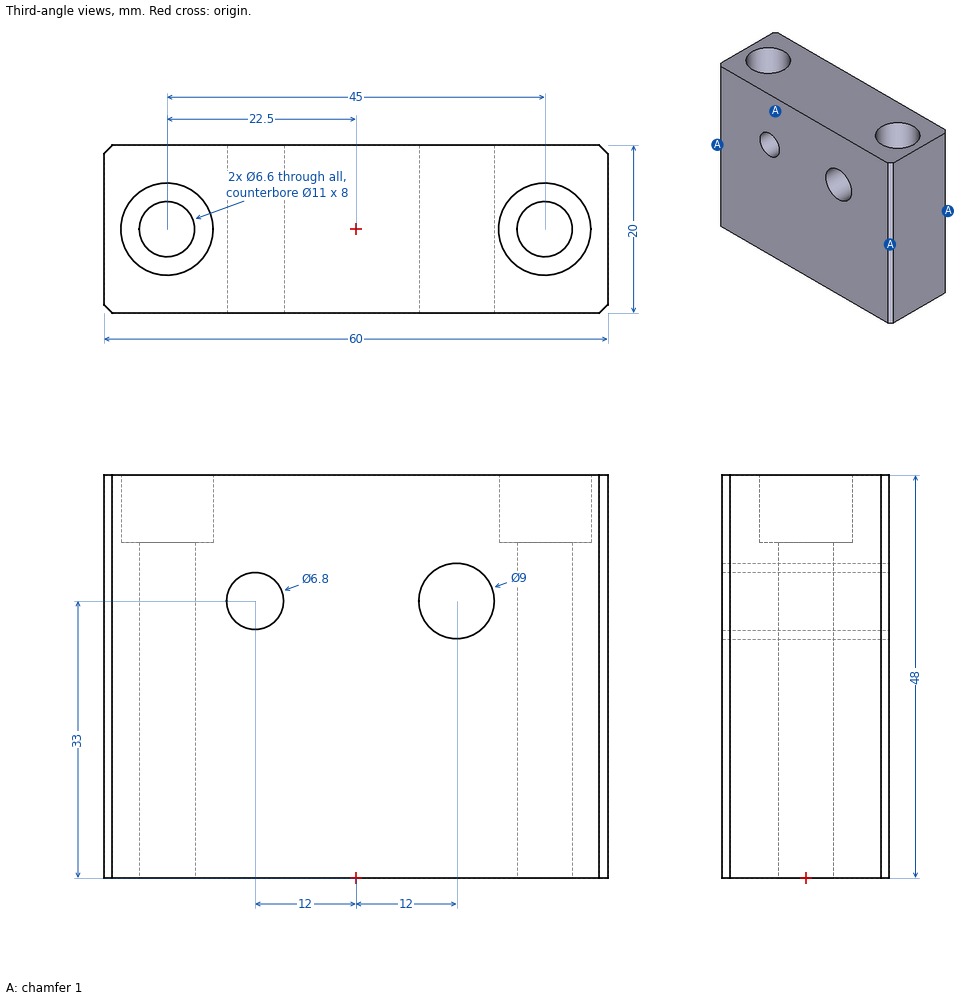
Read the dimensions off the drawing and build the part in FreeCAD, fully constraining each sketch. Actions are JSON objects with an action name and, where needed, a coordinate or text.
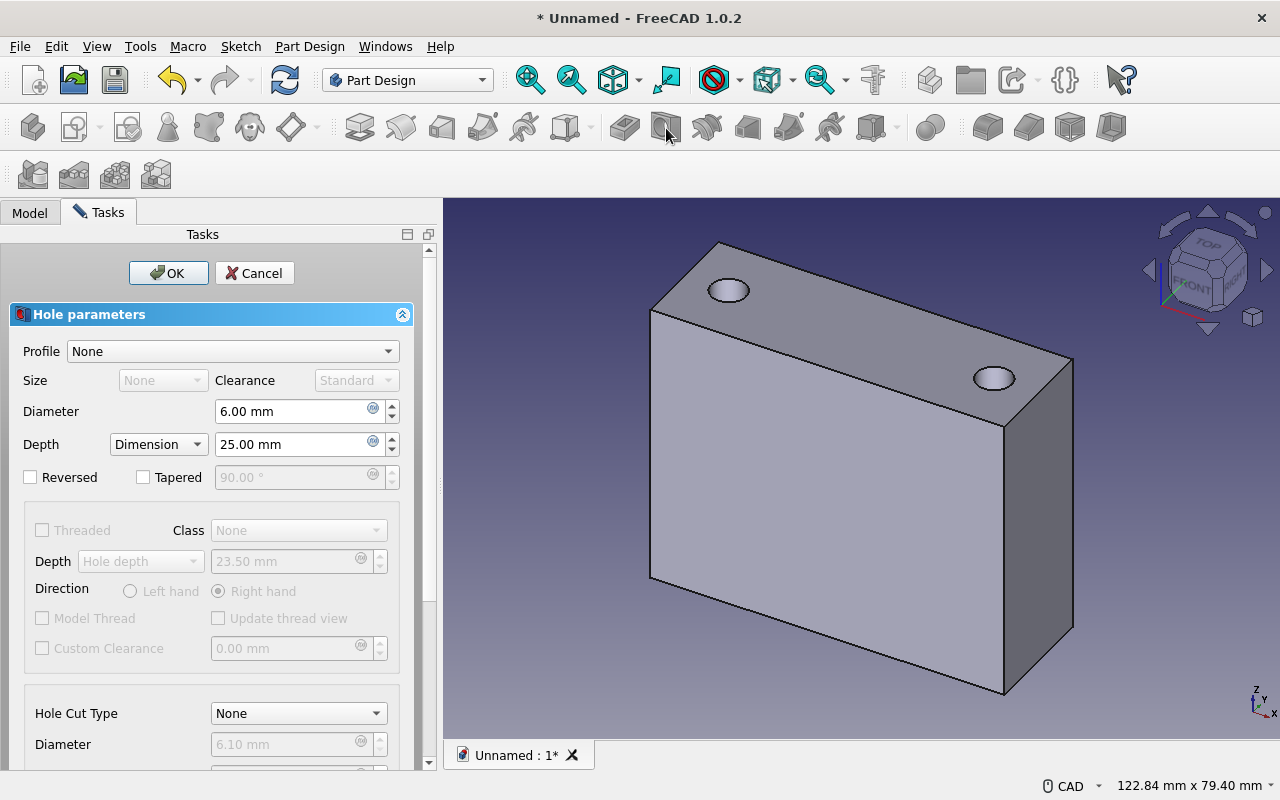
{"action": "triple_click", "coordinate": [300, 412]}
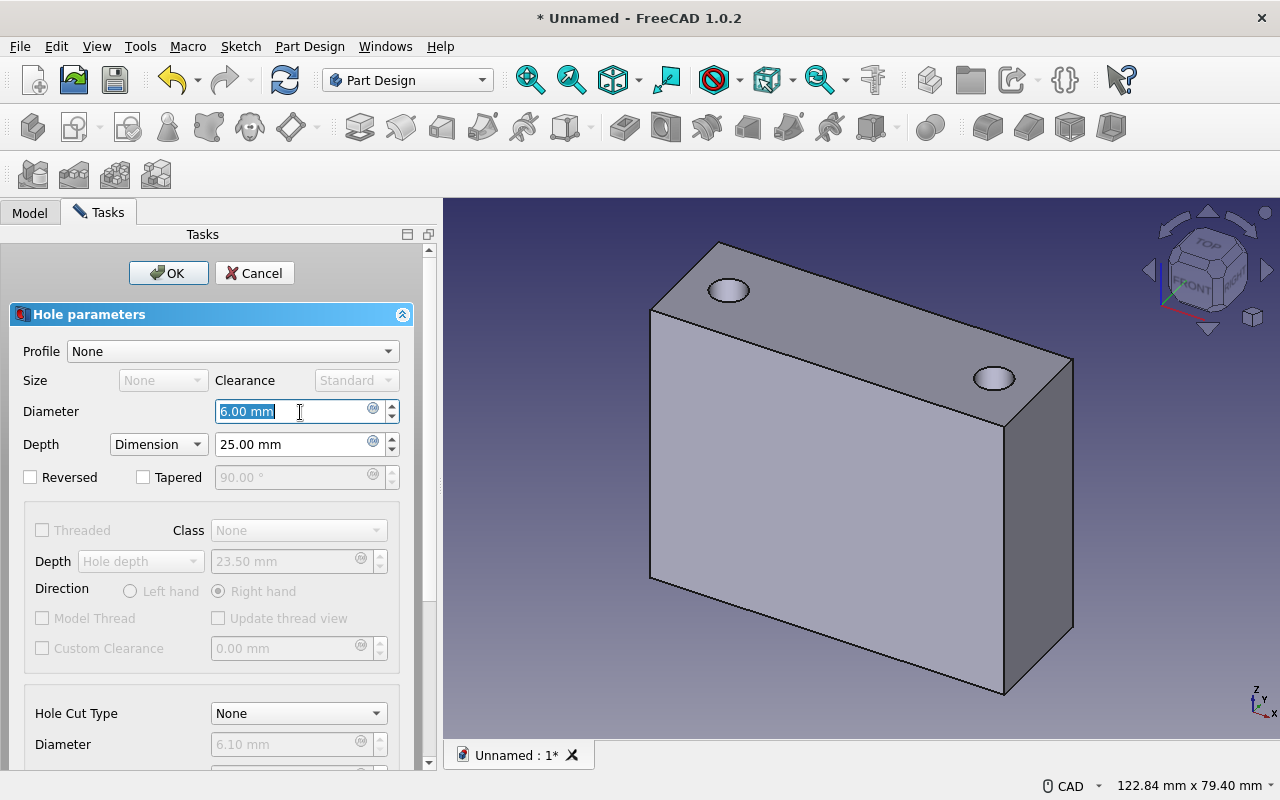
{"action": "type", "text": "6.6"}
{"action": "key", "text": "Tab"}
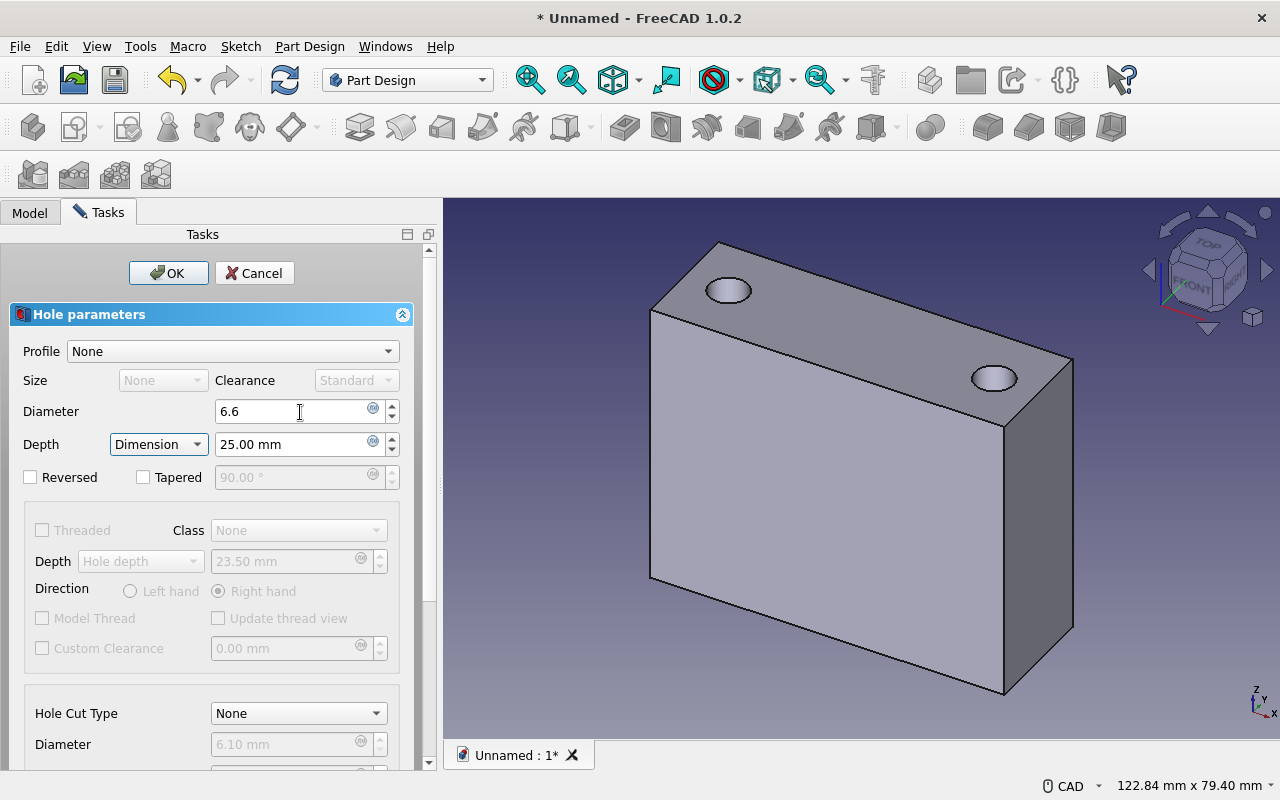
{"action": "left_click", "coordinate": [160, 444]}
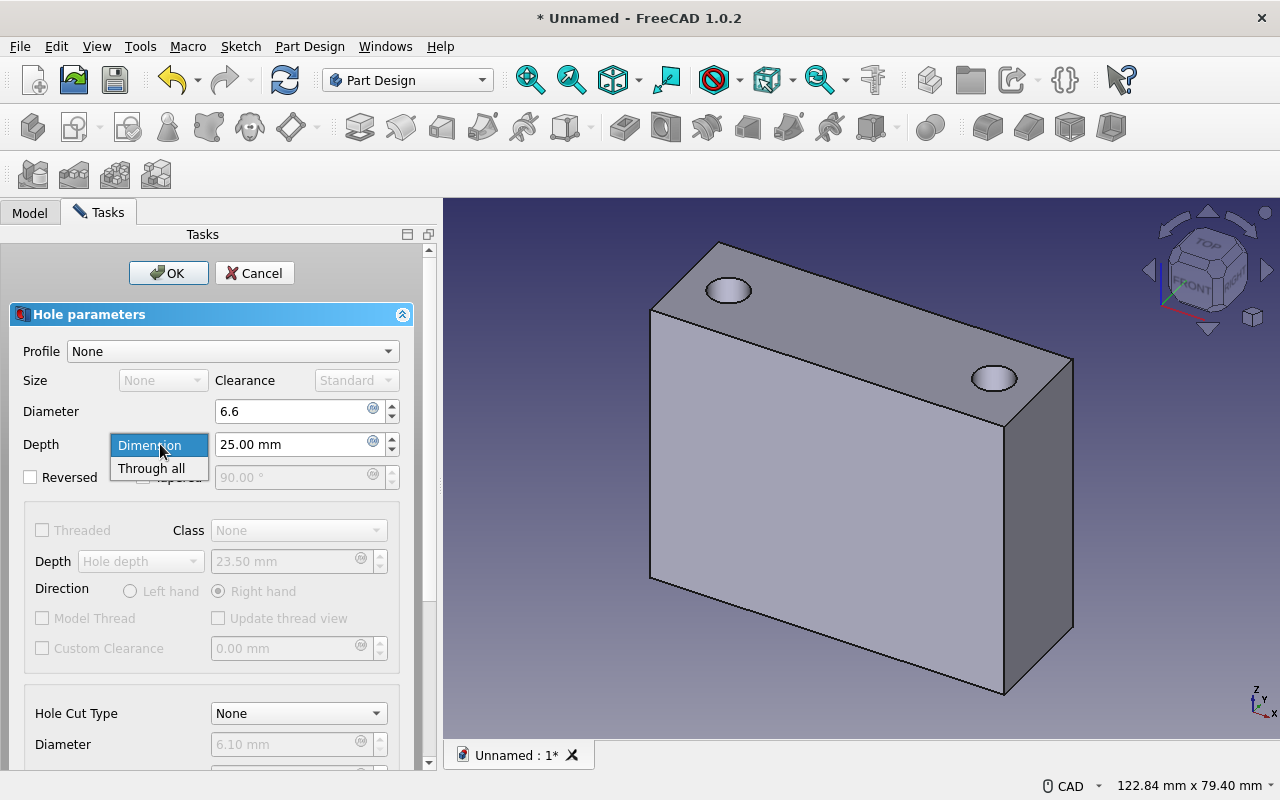
{"action": "left_click", "coordinate": [158, 468]}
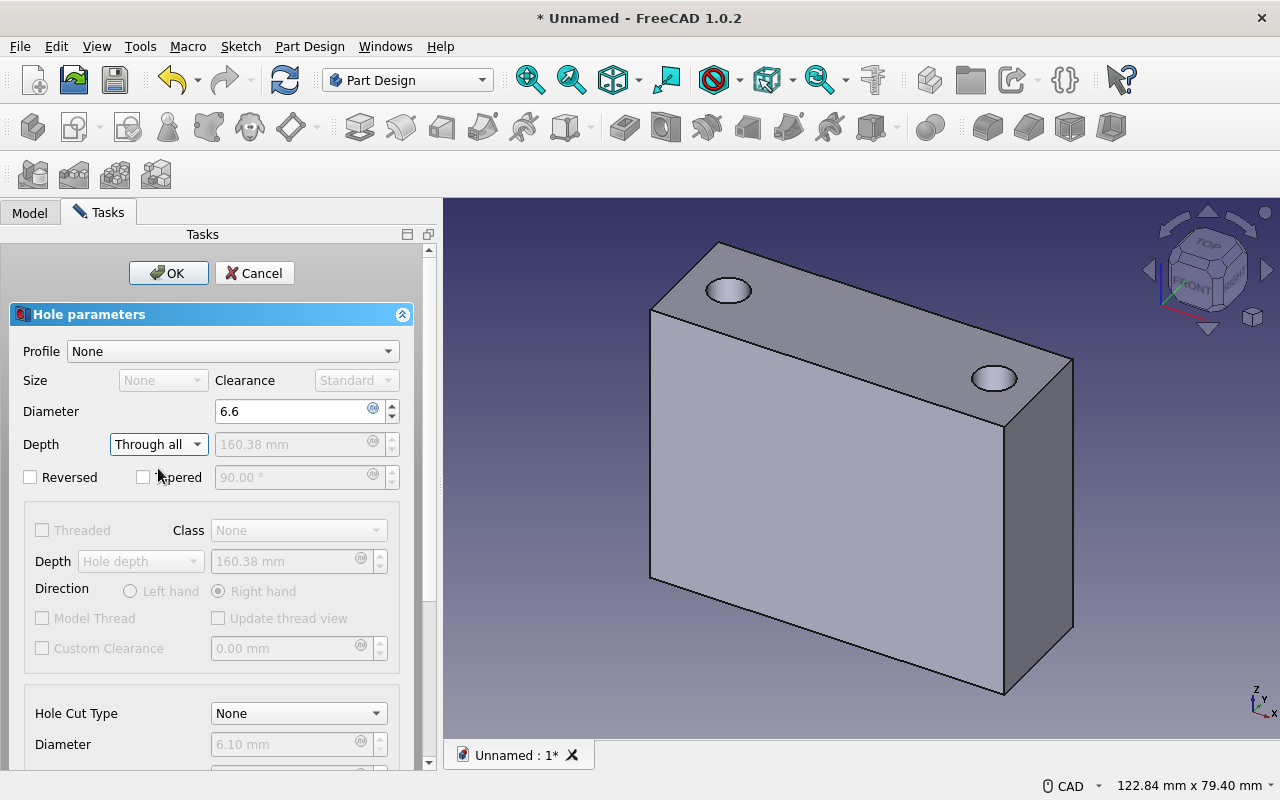
{"action": "left_click", "coordinate": [300, 714]}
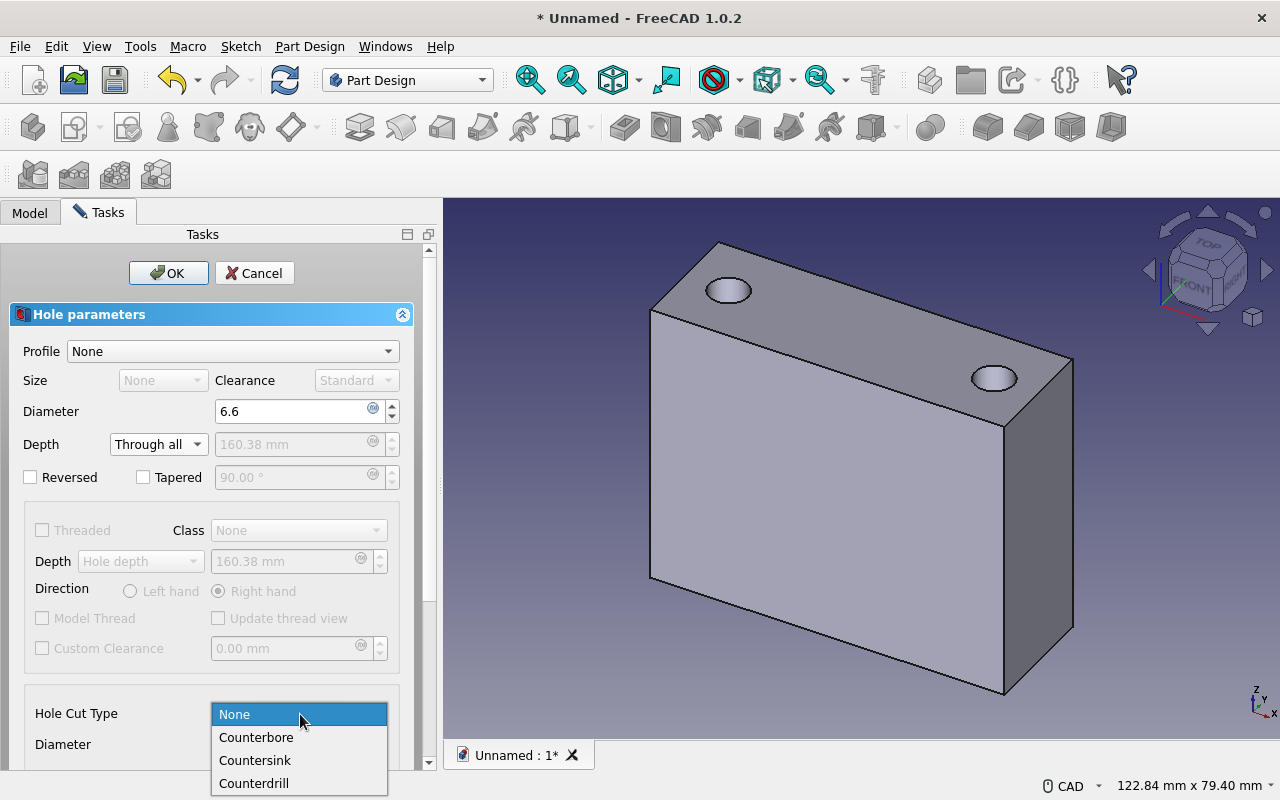
{"action": "left_click", "coordinate": [298, 738]}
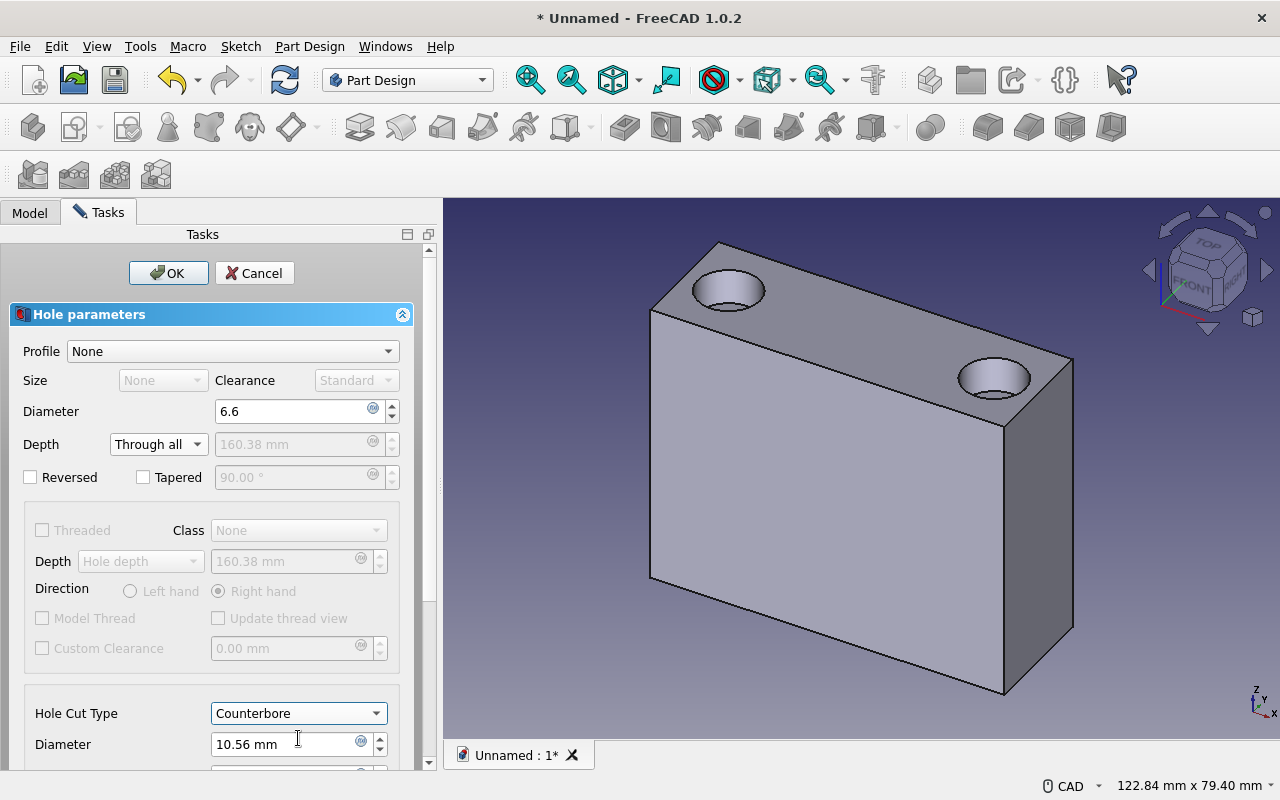
{"action": "triple_click", "coordinate": [292, 744]}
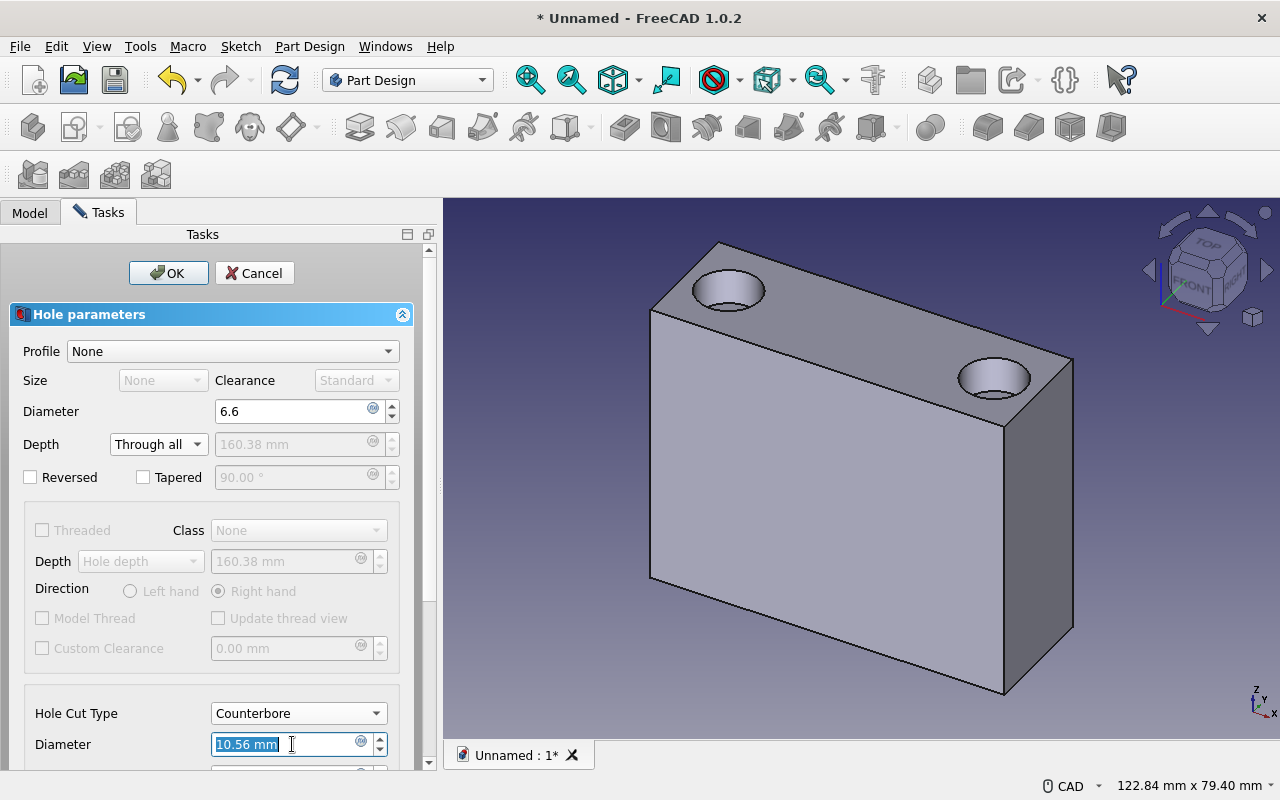
{"action": "type", "text": "11"}
{"action": "key", "text": "Tab"}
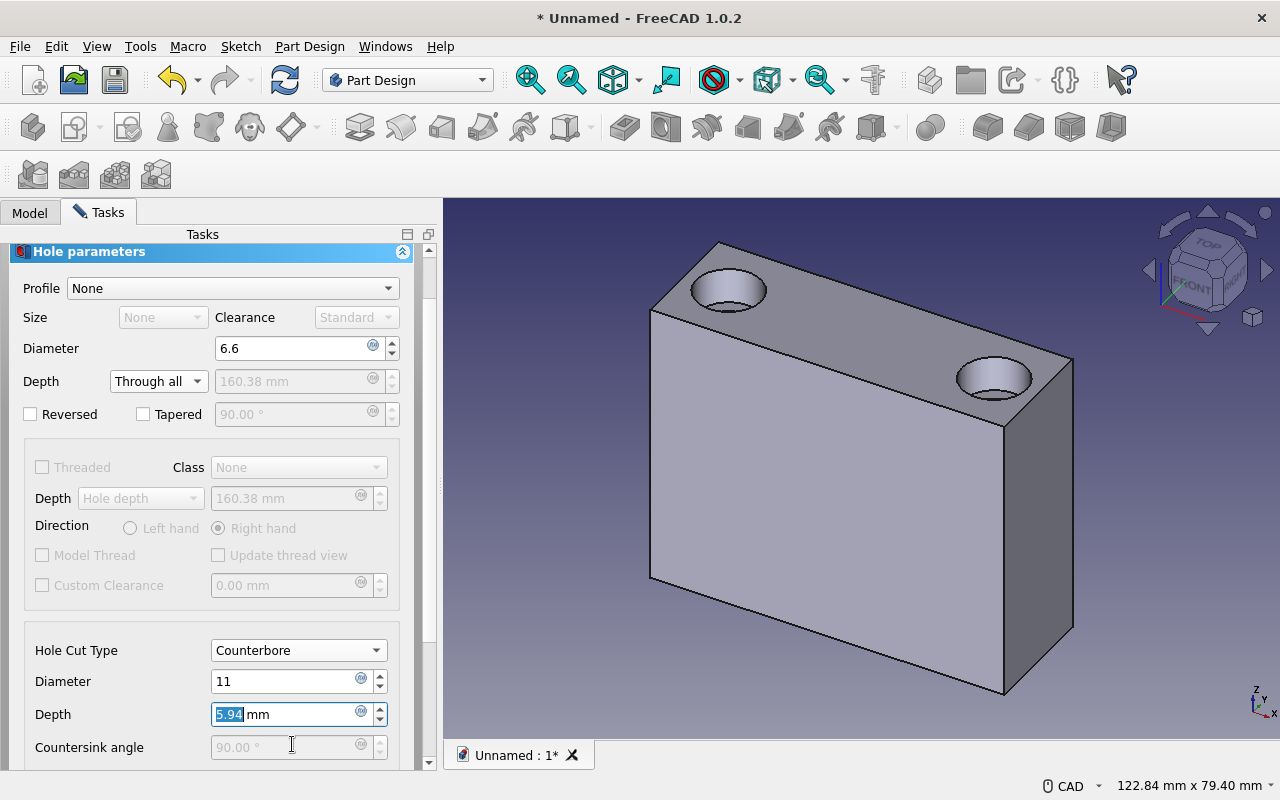
{"action": "type", "text": "8"}
{"action": "key", "text": "Tab"}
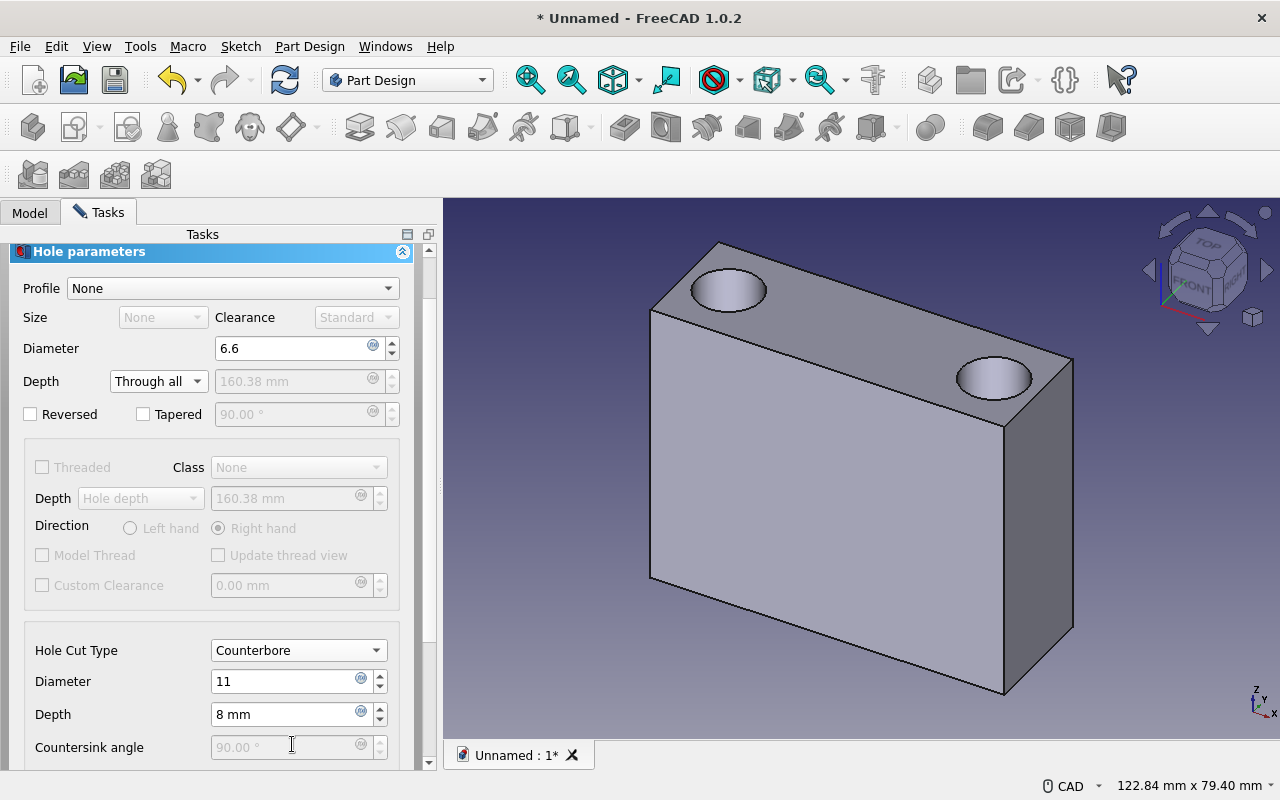
{"action": "scroll", "coordinate": [429, 507], "scroll_direction": "up", "scroll_amount": 2}